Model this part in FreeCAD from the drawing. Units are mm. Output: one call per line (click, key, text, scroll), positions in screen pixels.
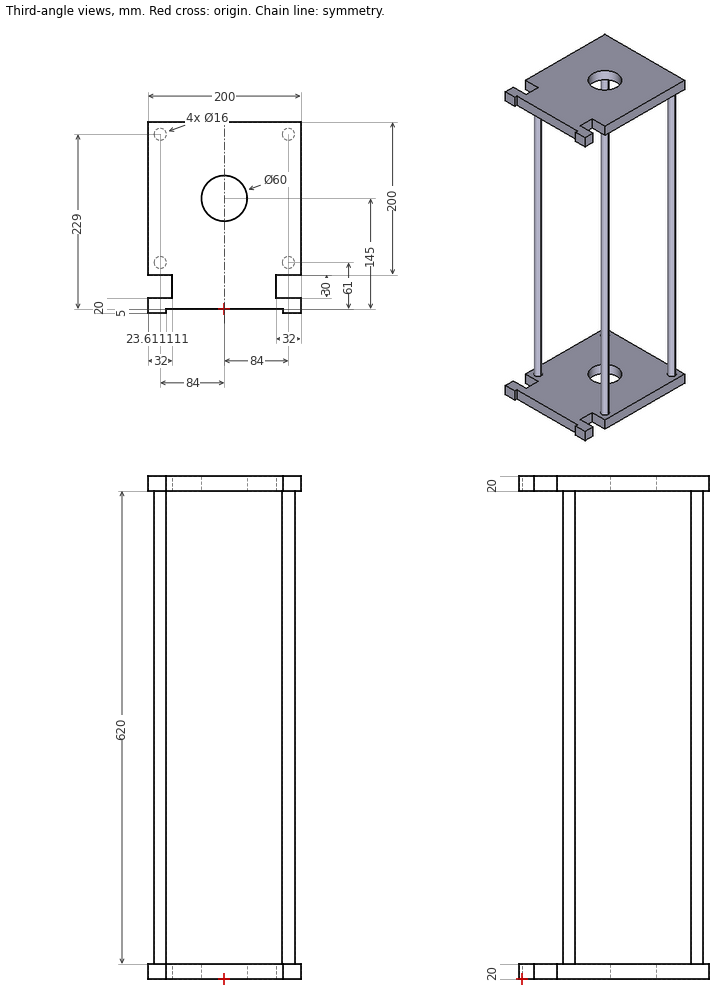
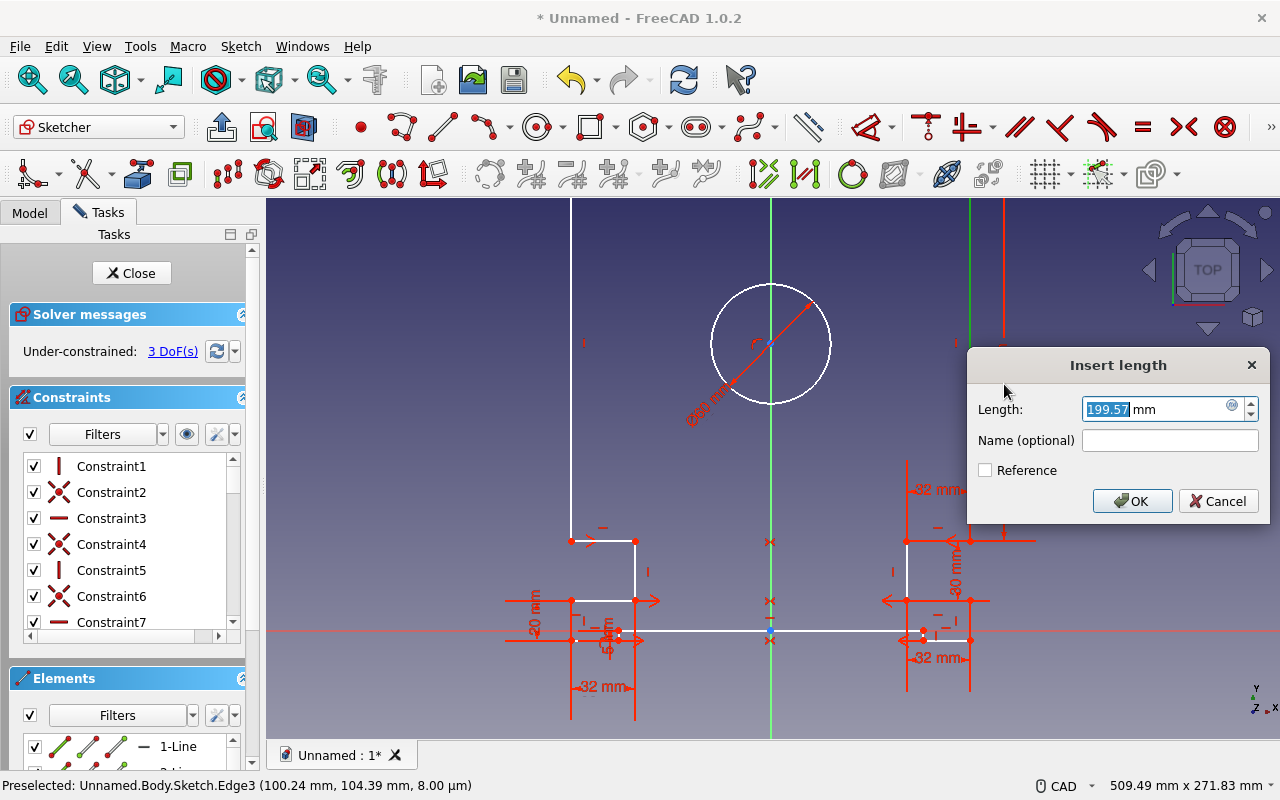
text(200)
key(Return)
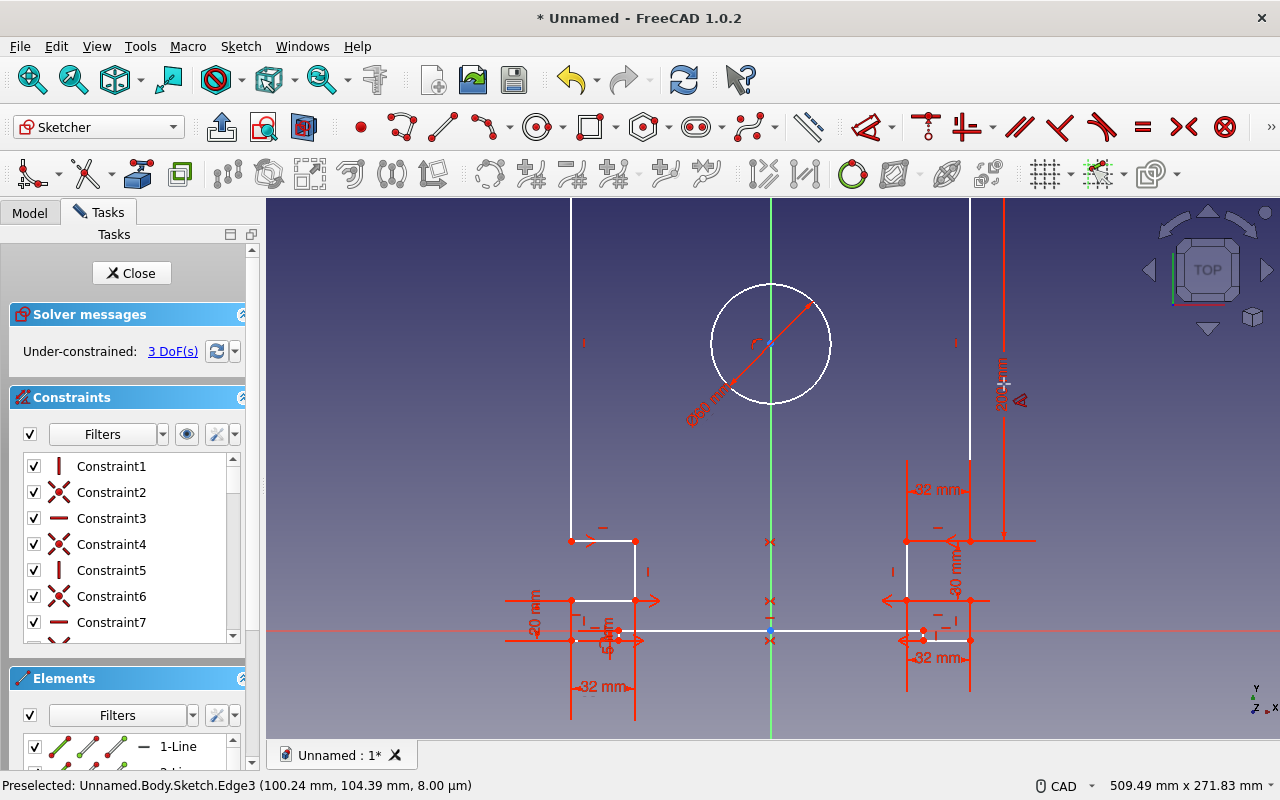
scroll(569, 624, down, 2)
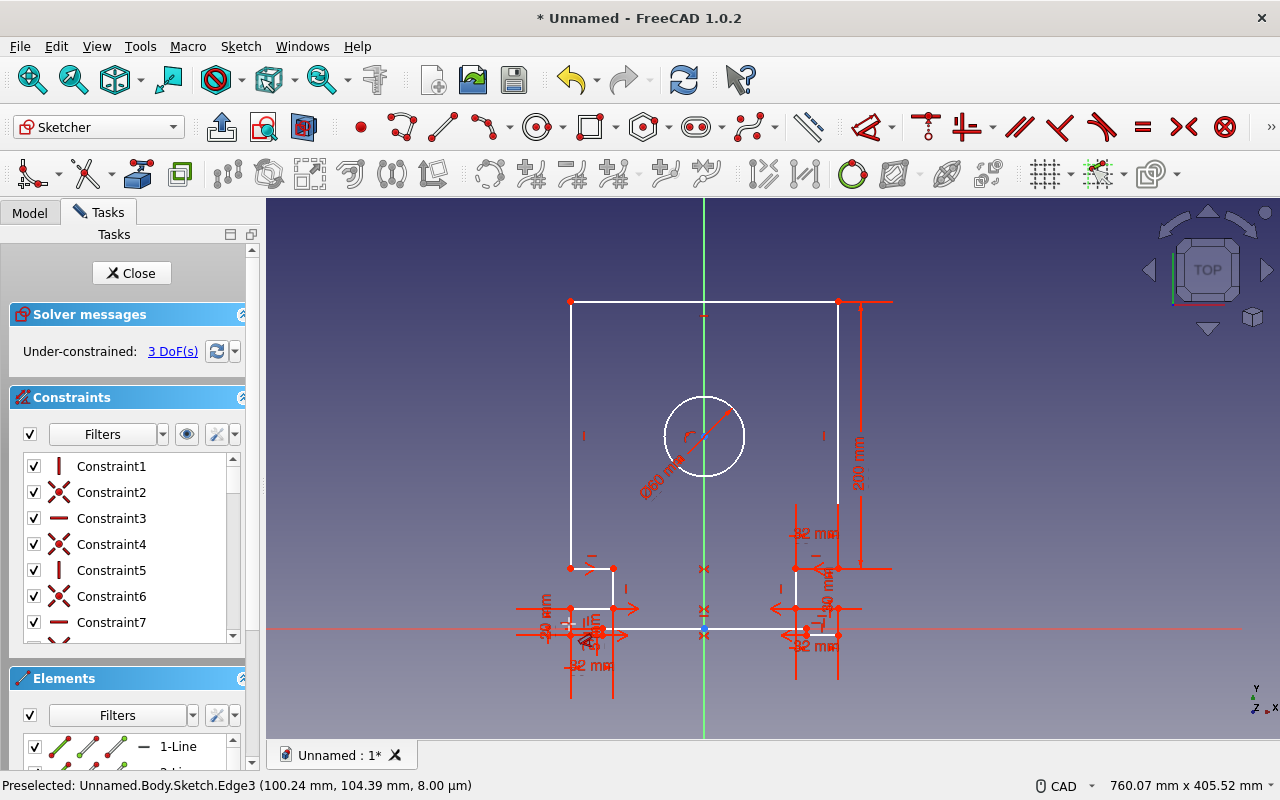
click(758, 302)
click(643, 268)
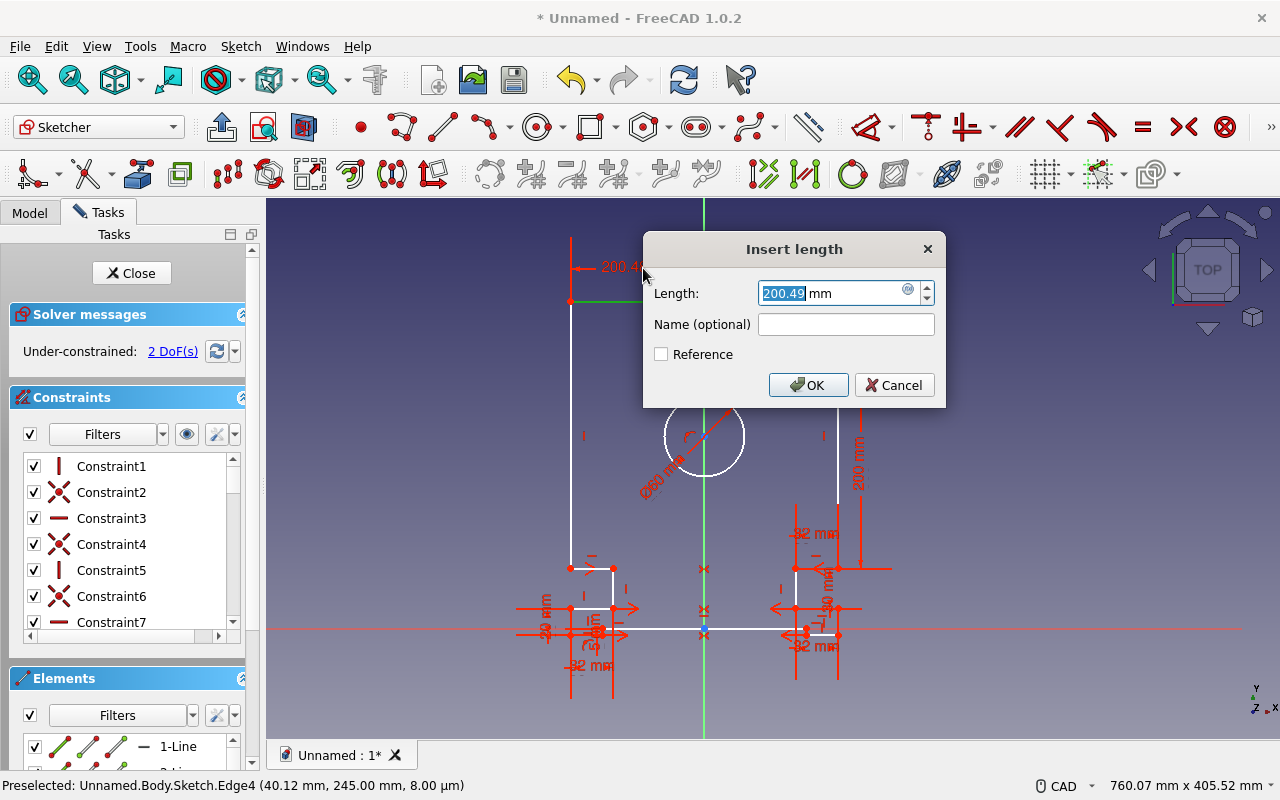
text(200)
key(Return)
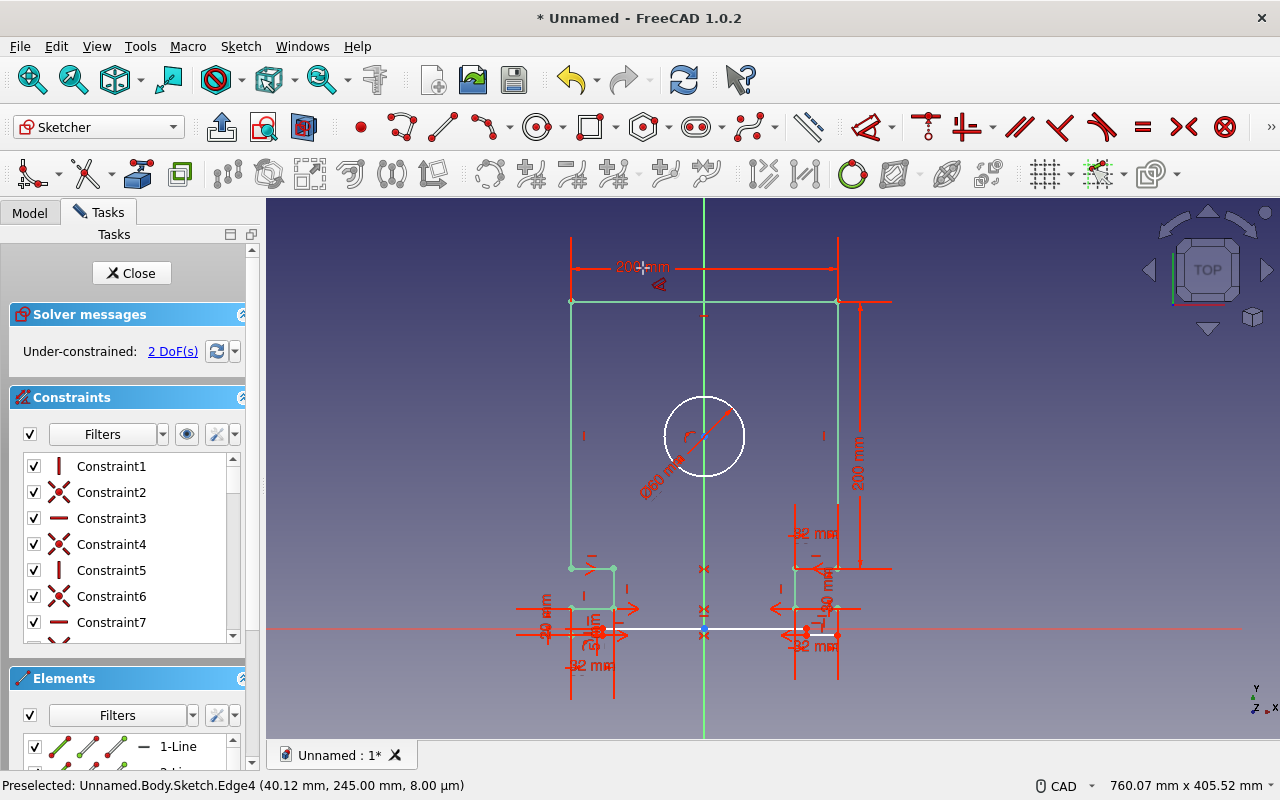
click(704, 437)
click(738, 533)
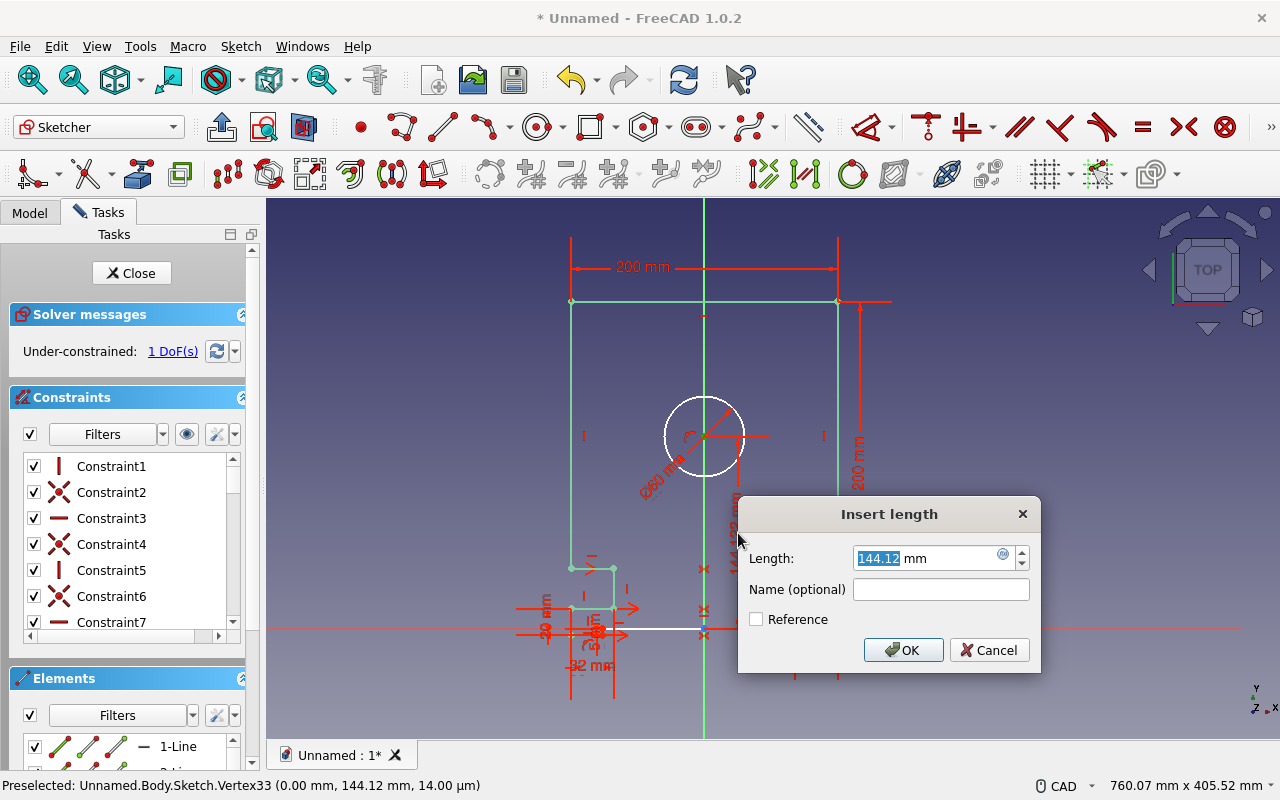
text(145)
key(Return)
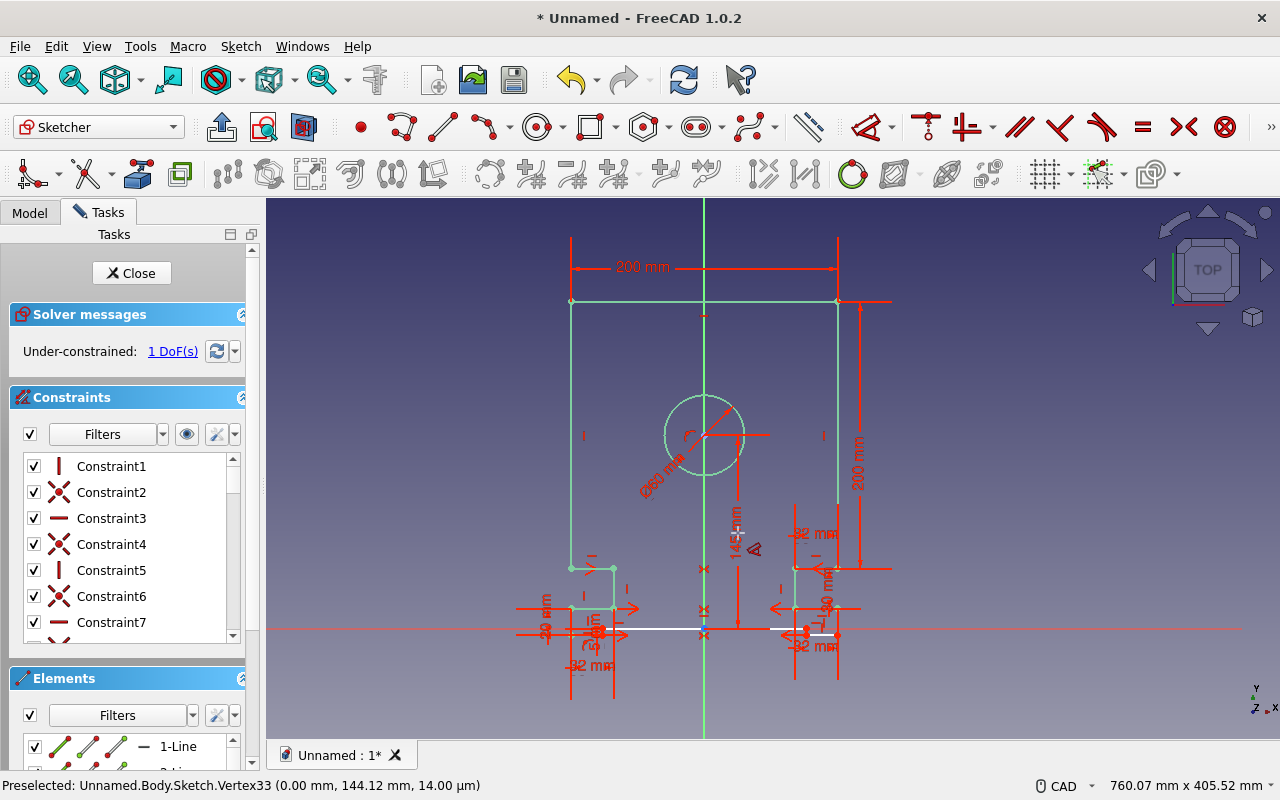
scroll(580, 635, up, 4)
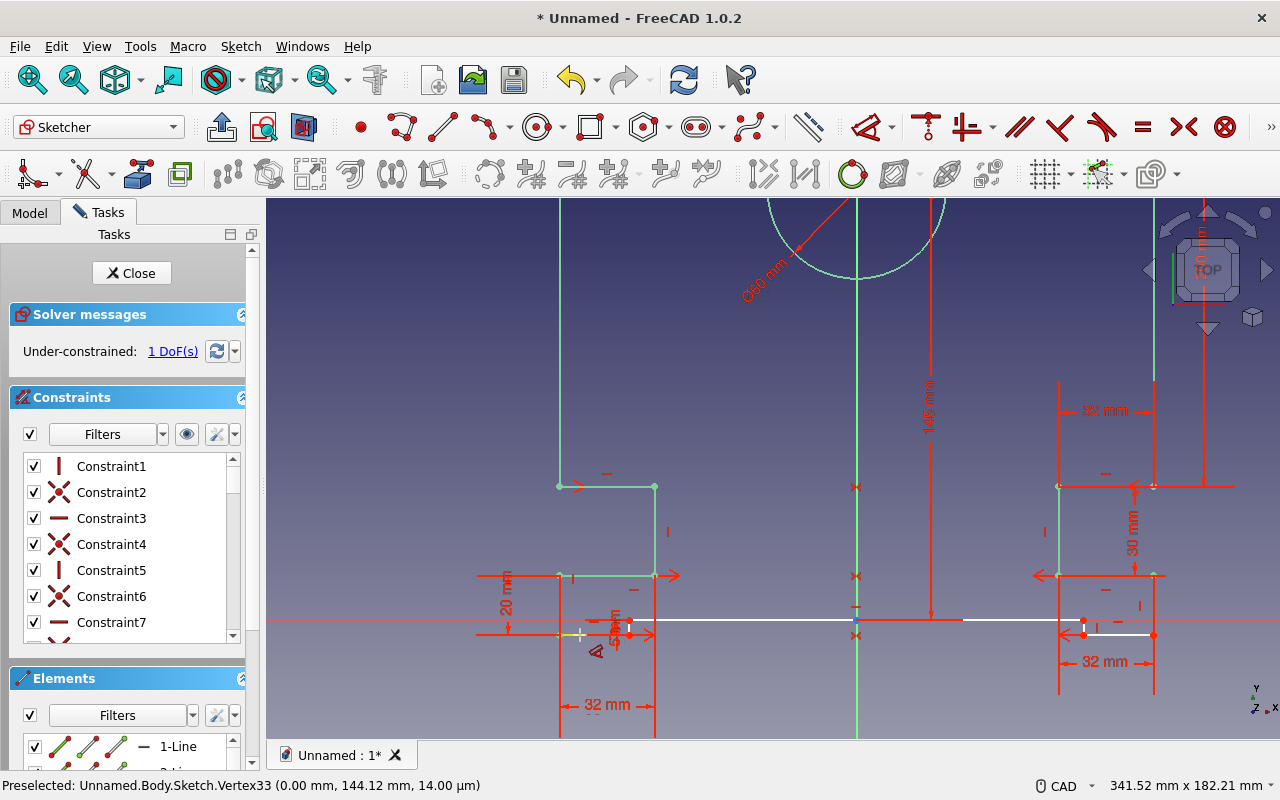
click(581, 635)
click(595, 669)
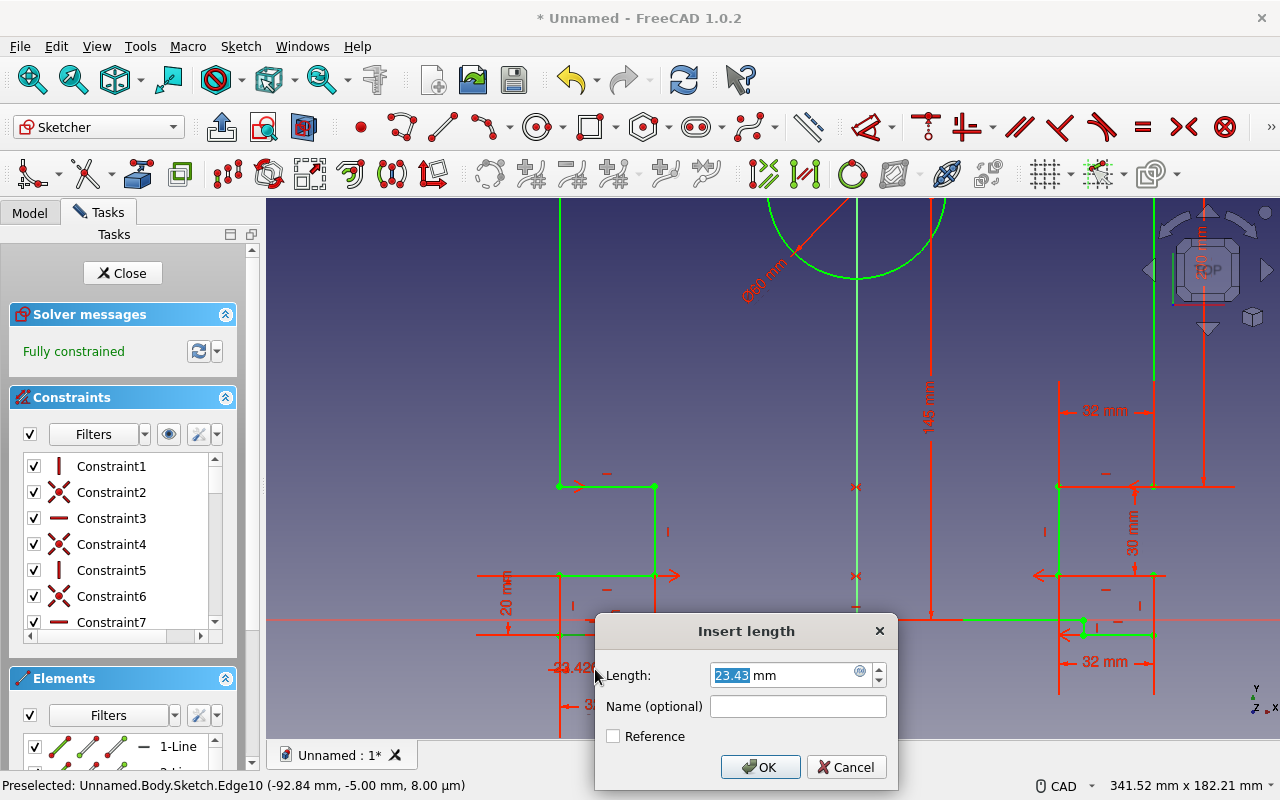
text(23.611111)
key(Return)
key(Escape)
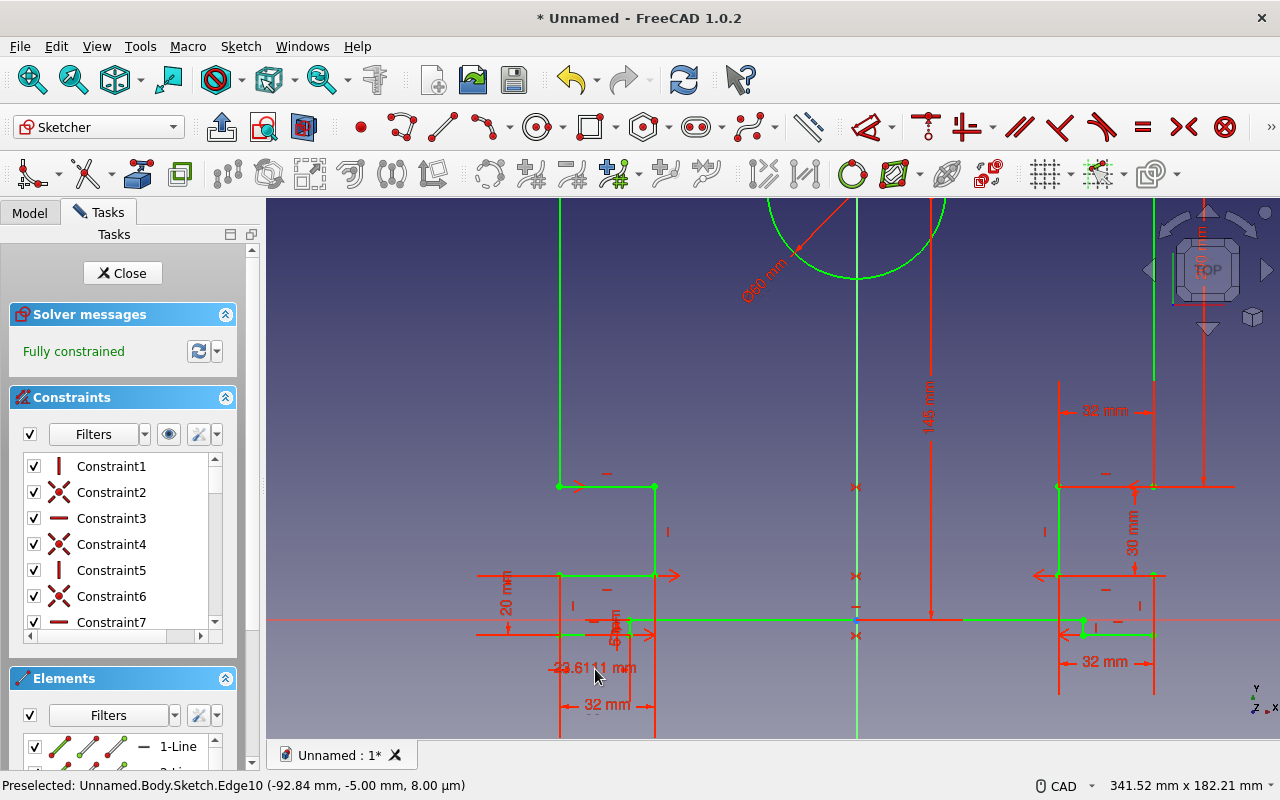
click(123, 273)